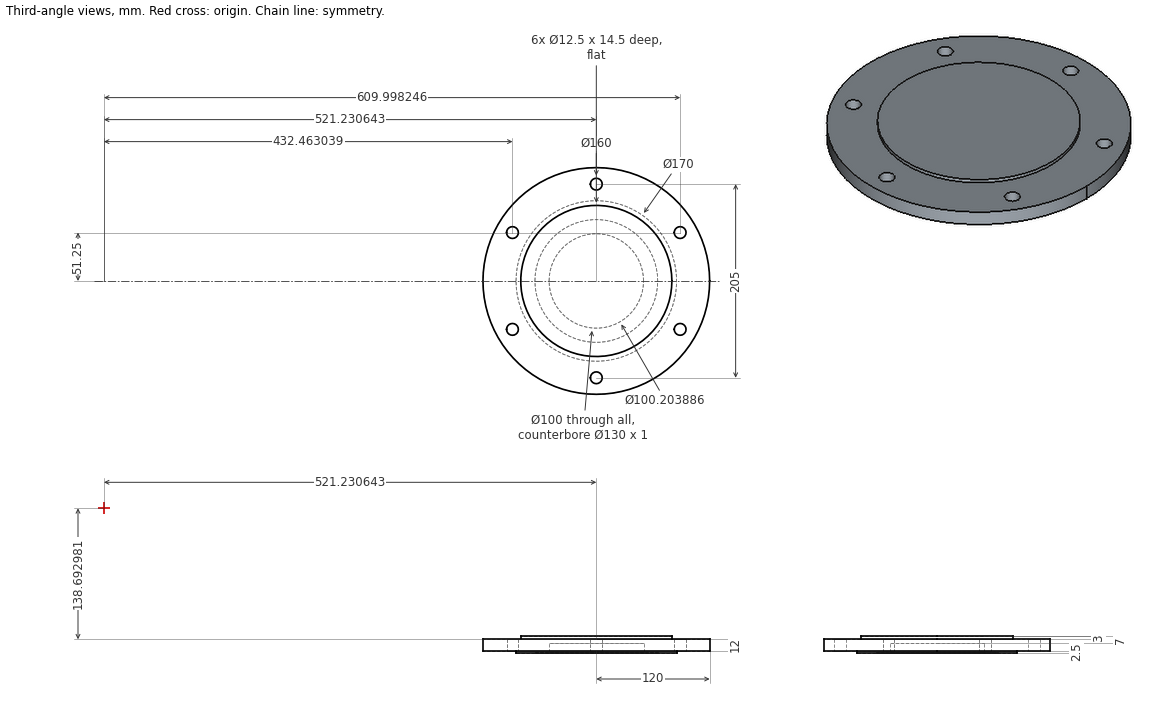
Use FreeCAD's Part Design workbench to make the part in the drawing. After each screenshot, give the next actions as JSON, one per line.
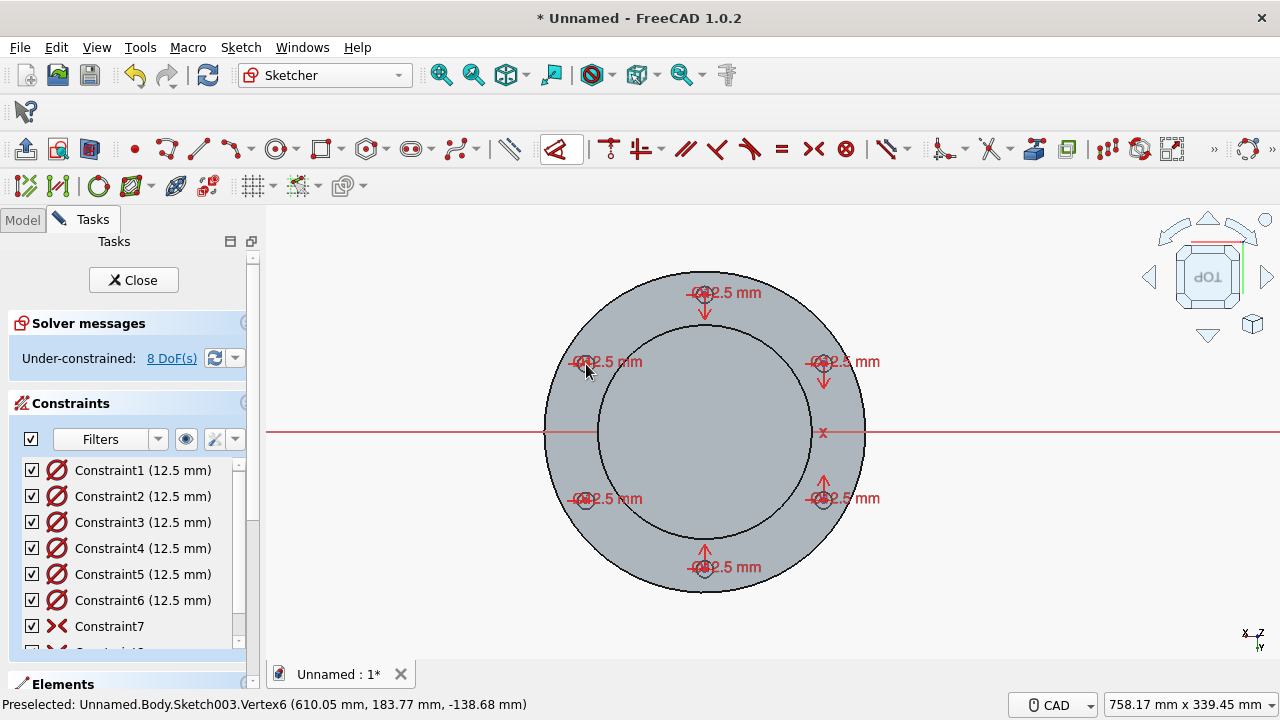
{"action": "left_click", "coordinate": [353, 432]}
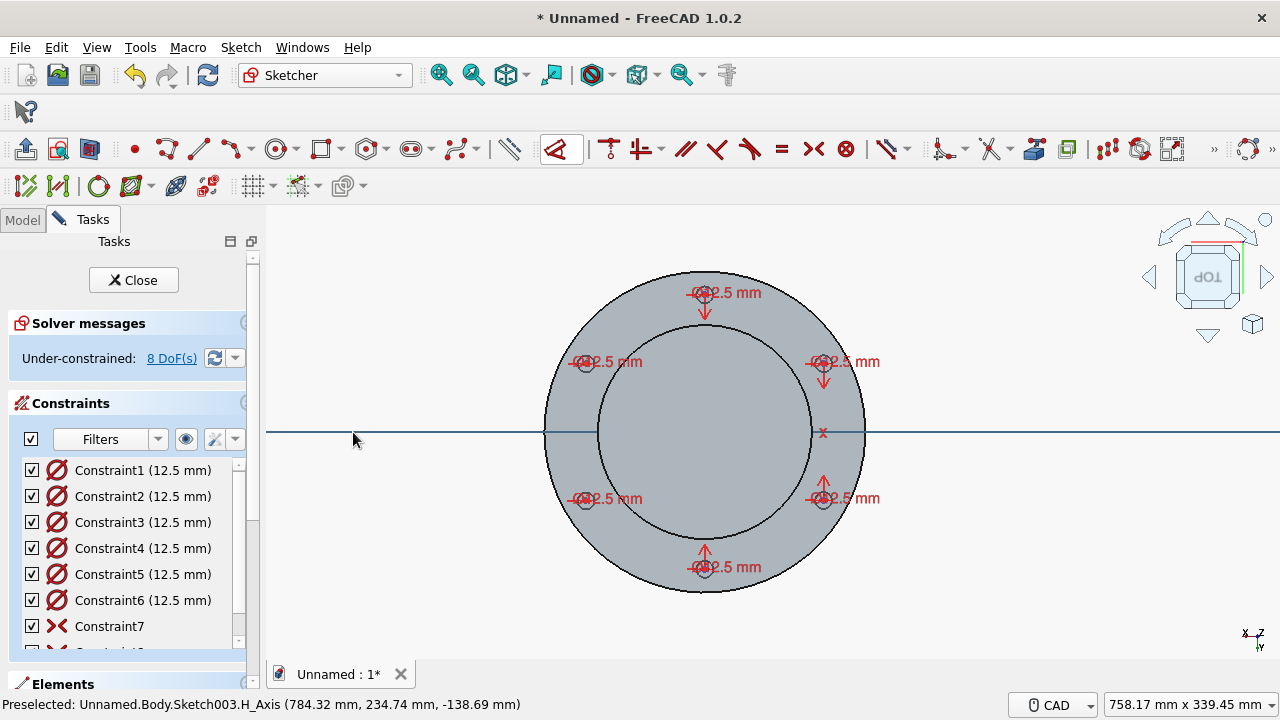
{"action": "key", "text": "s"}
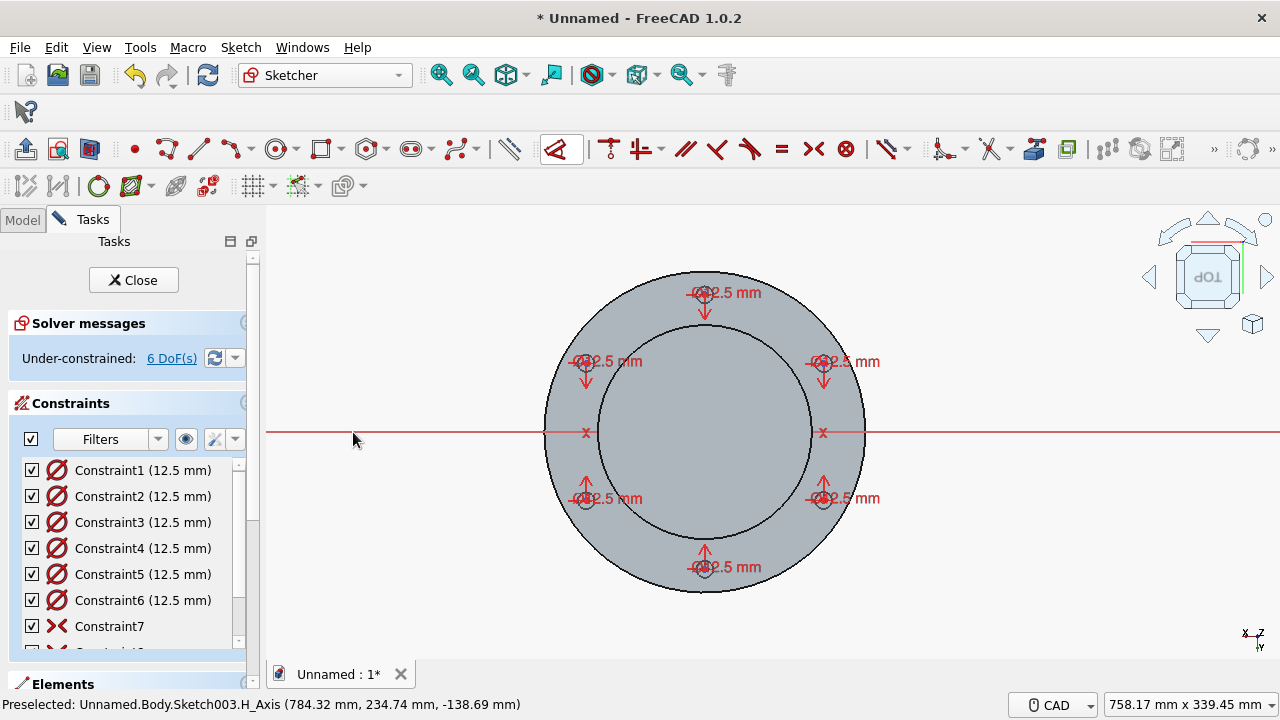
{"action": "left_click", "coordinate": [556, 150]}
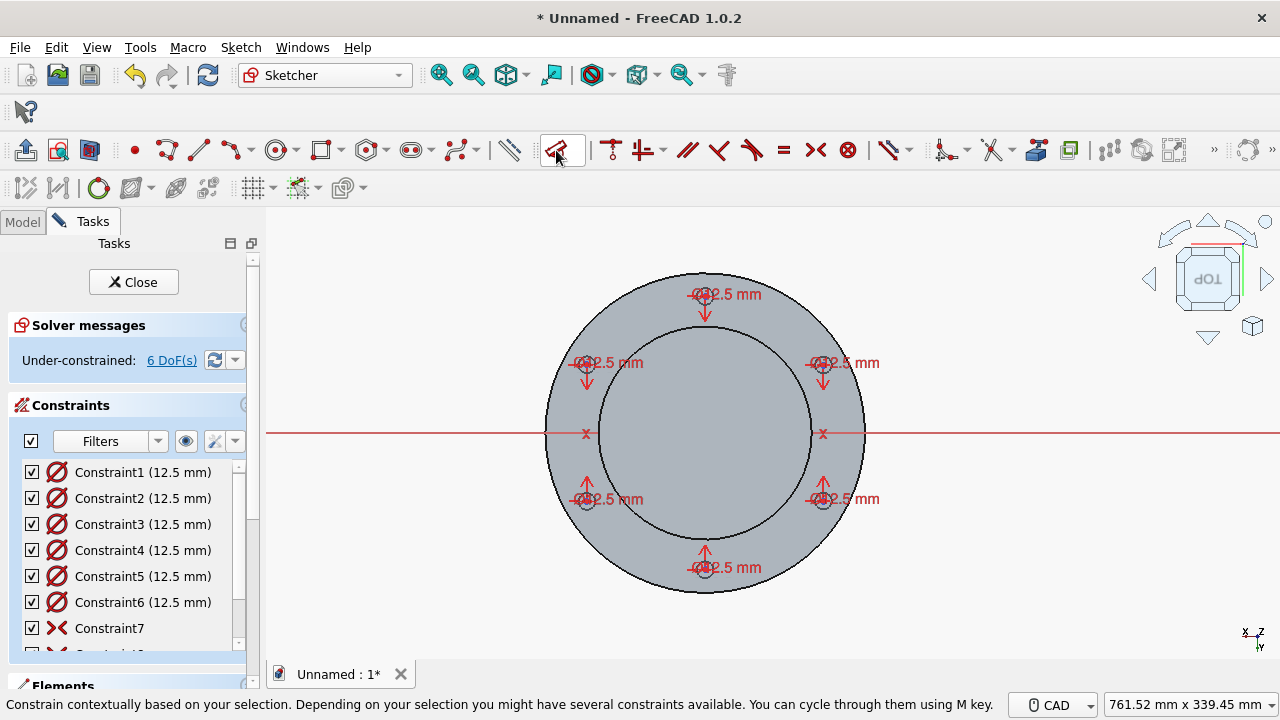
{"action": "left_click", "coordinate": [705, 570]}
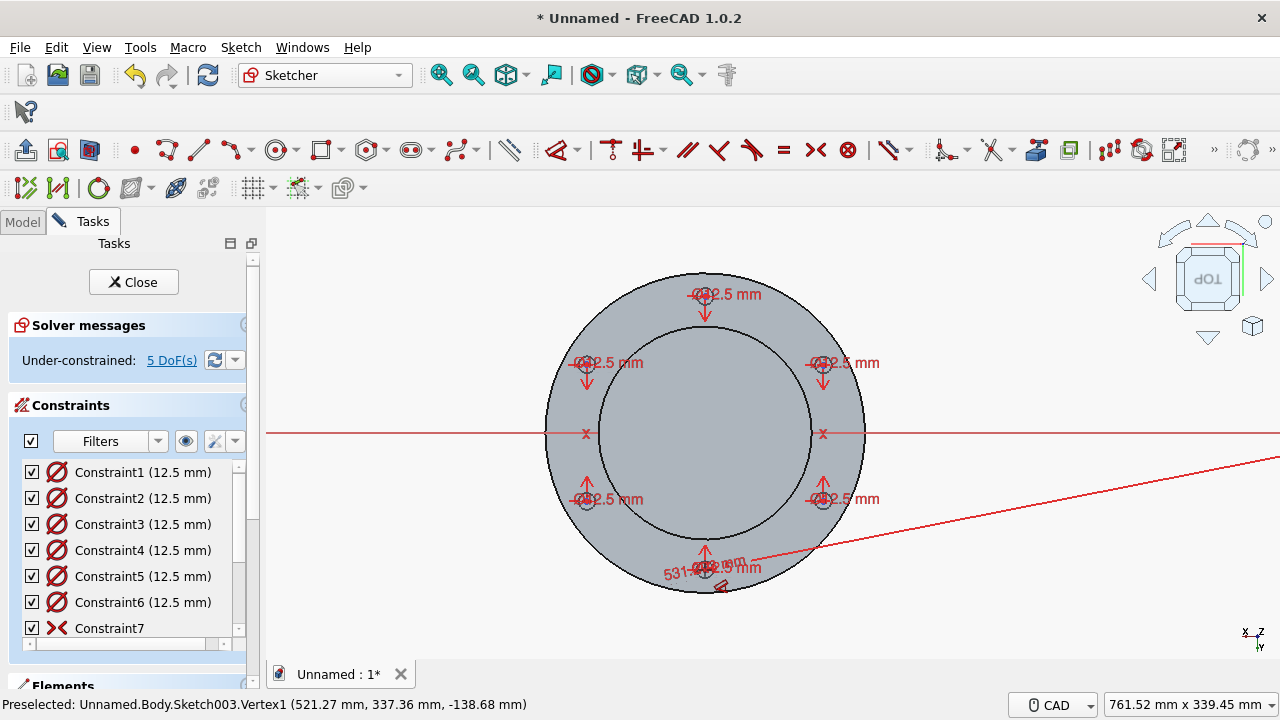
{"action": "left_click", "coordinate": [705, 296]}
{"action": "left_click", "coordinate": [671, 370]}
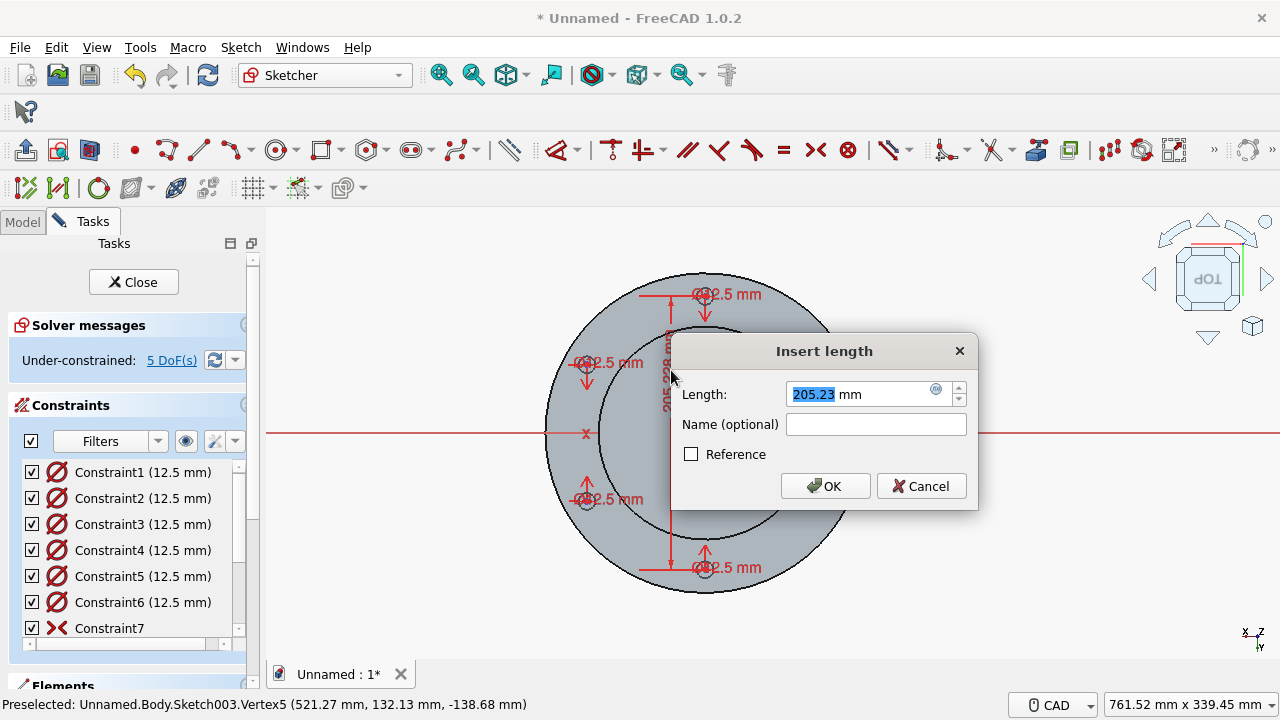
{"action": "type", "text": "205"}
{"action": "key", "text": "Return"}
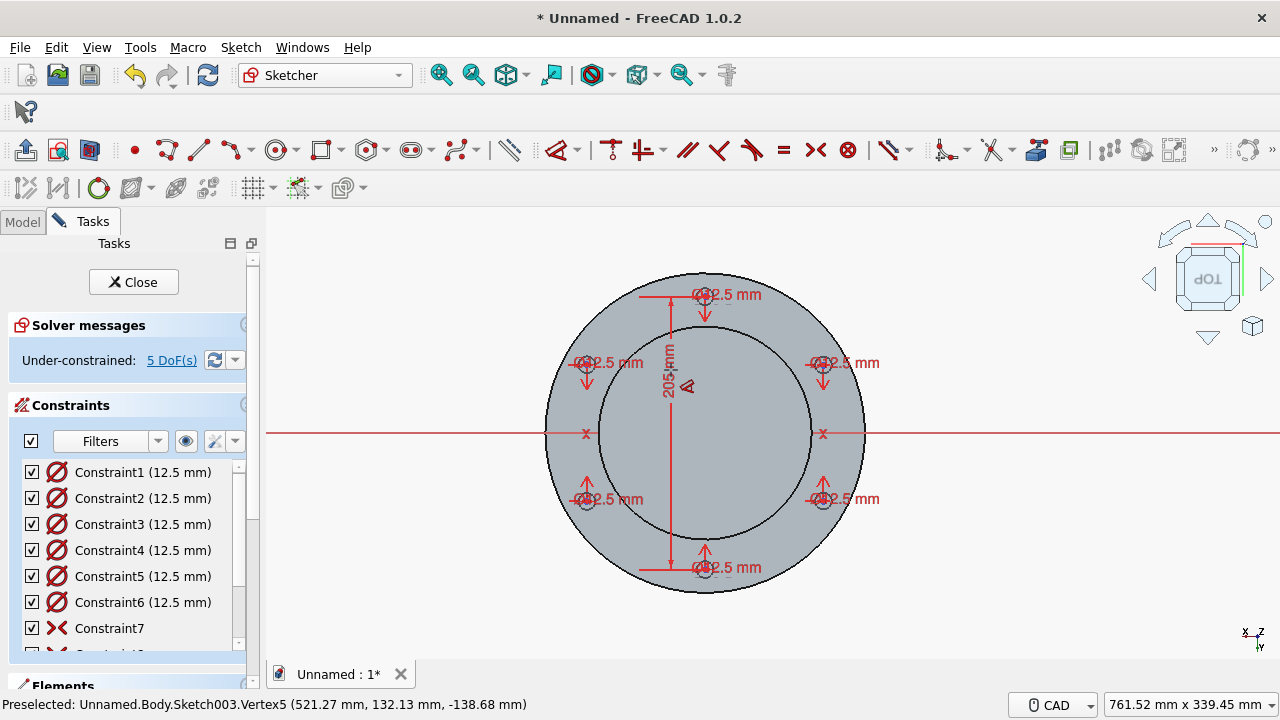
{"action": "left_click", "coordinate": [587, 501]}
{"action": "left_click", "coordinate": [553, 467]}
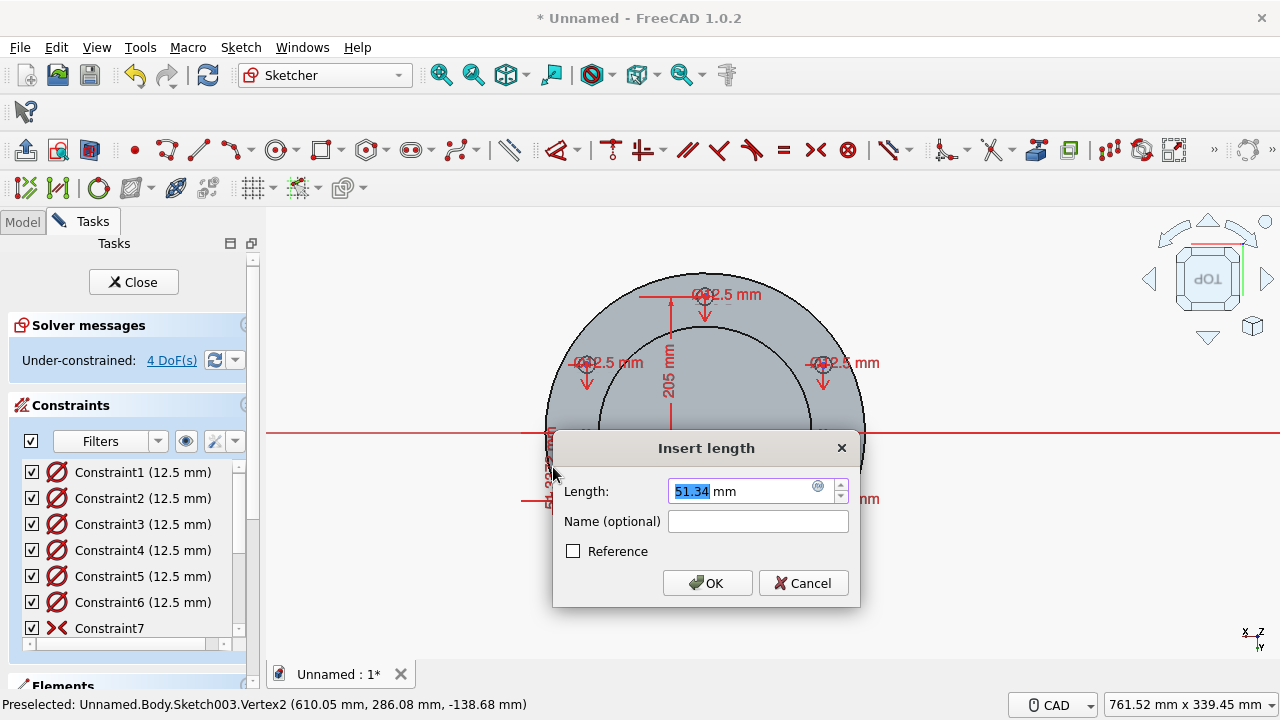
{"action": "type", "text": "51.25"}
{"action": "key", "text": "Return"}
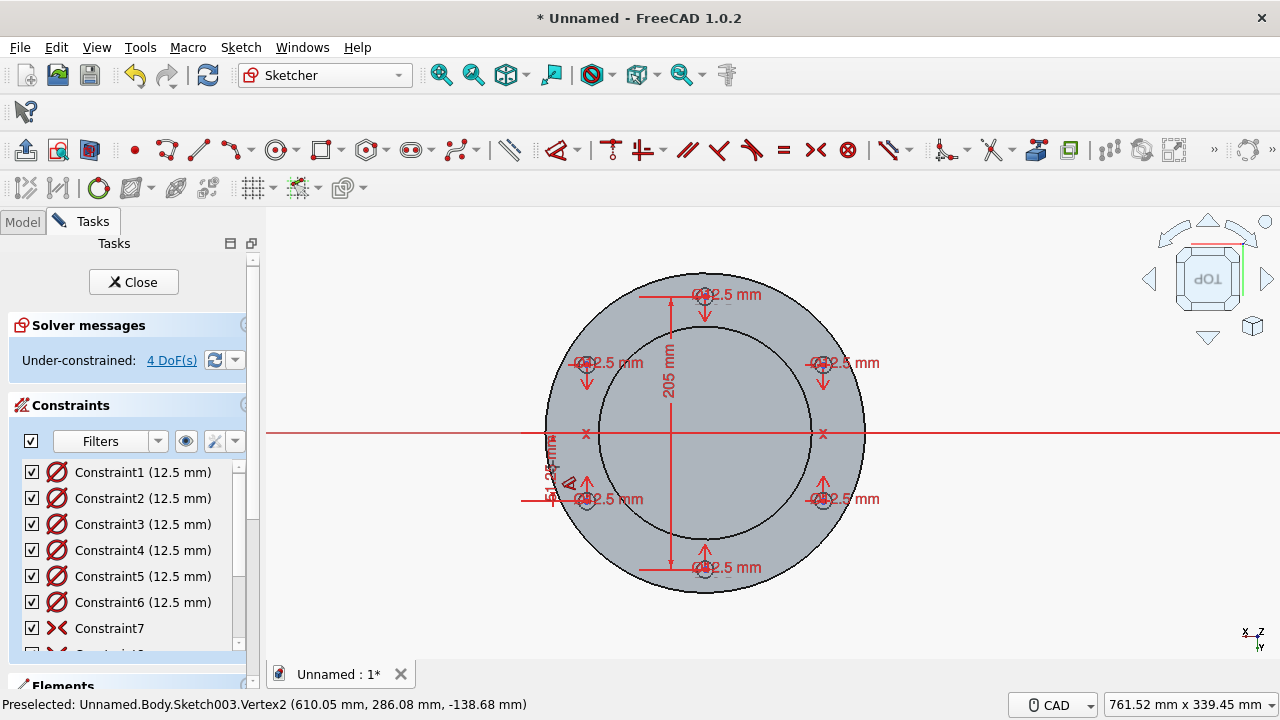
{"action": "left_click", "coordinate": [823, 501]}
{"action": "left_click", "coordinate": [789, 467]}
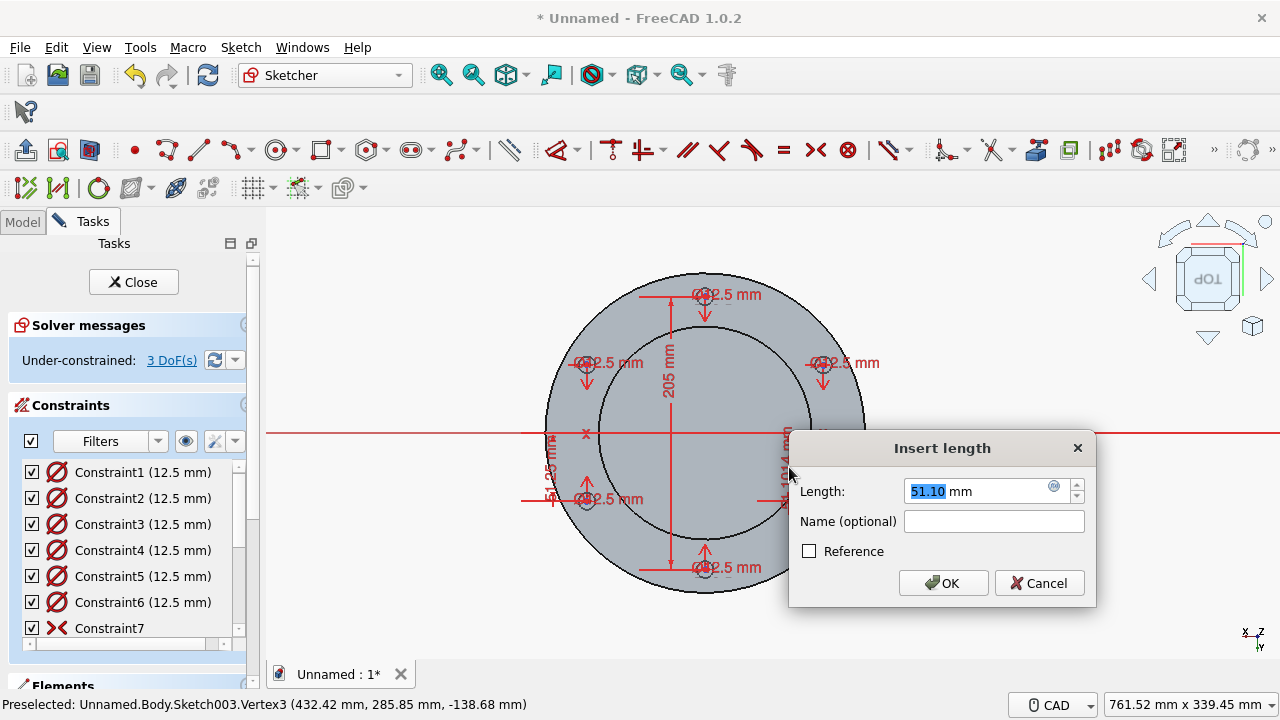
{"action": "type", "text": "51.25"}
{"action": "key", "text": "Return"}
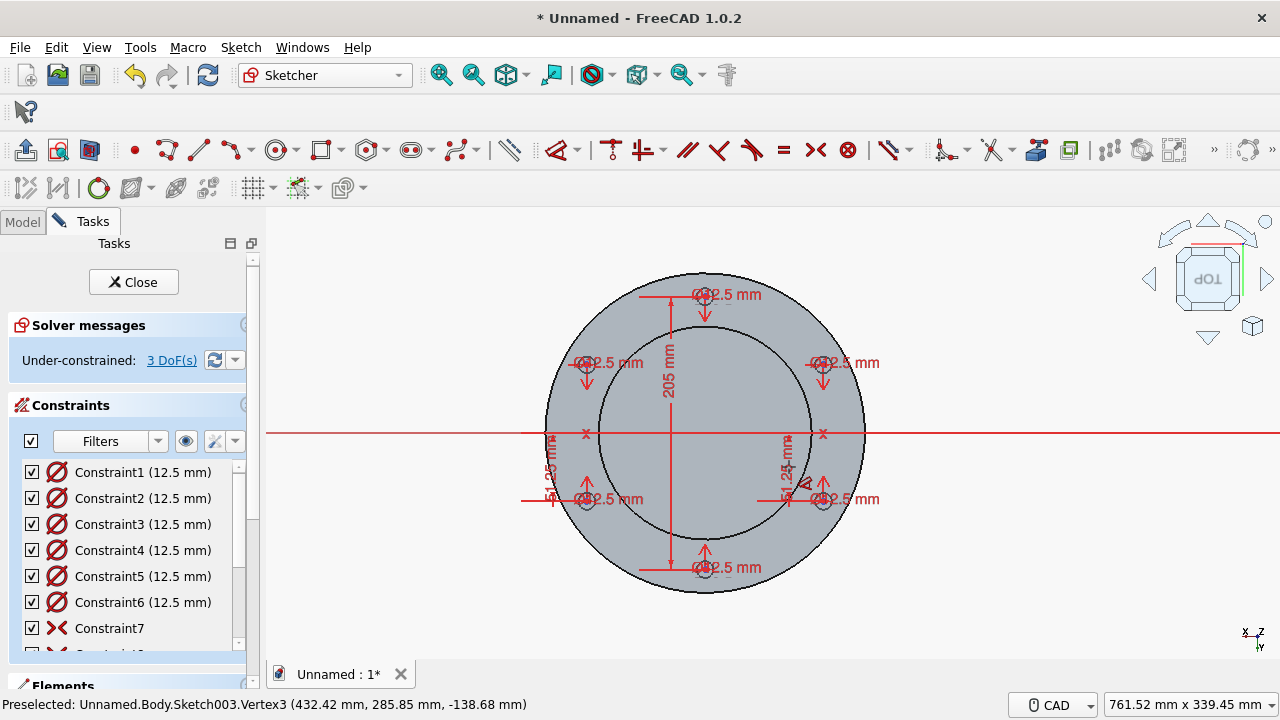
{"action": "left_click", "coordinate": [705, 570]}
{"action": "left_click", "coordinate": [910, 604]}